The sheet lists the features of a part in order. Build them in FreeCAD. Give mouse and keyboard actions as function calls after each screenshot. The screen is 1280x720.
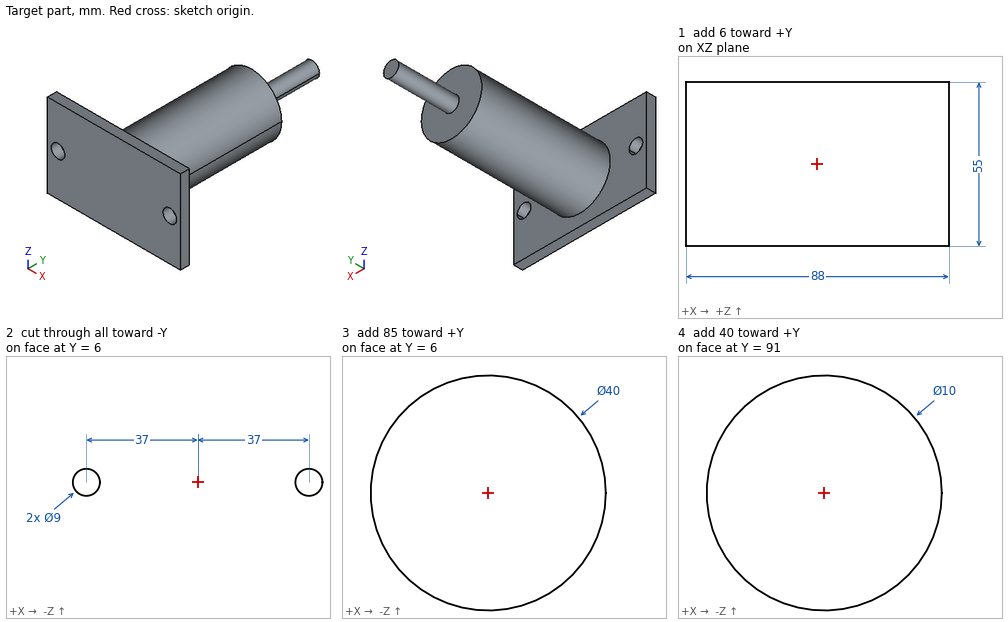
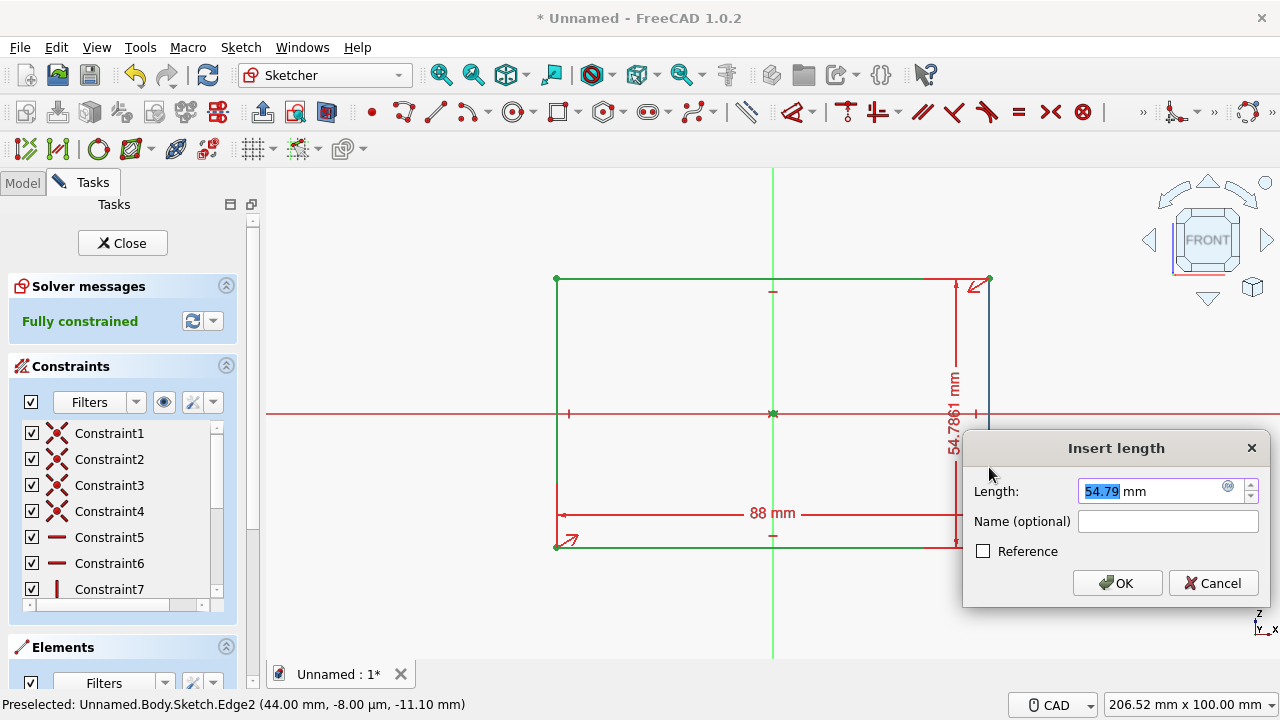
text(55)
key(Return)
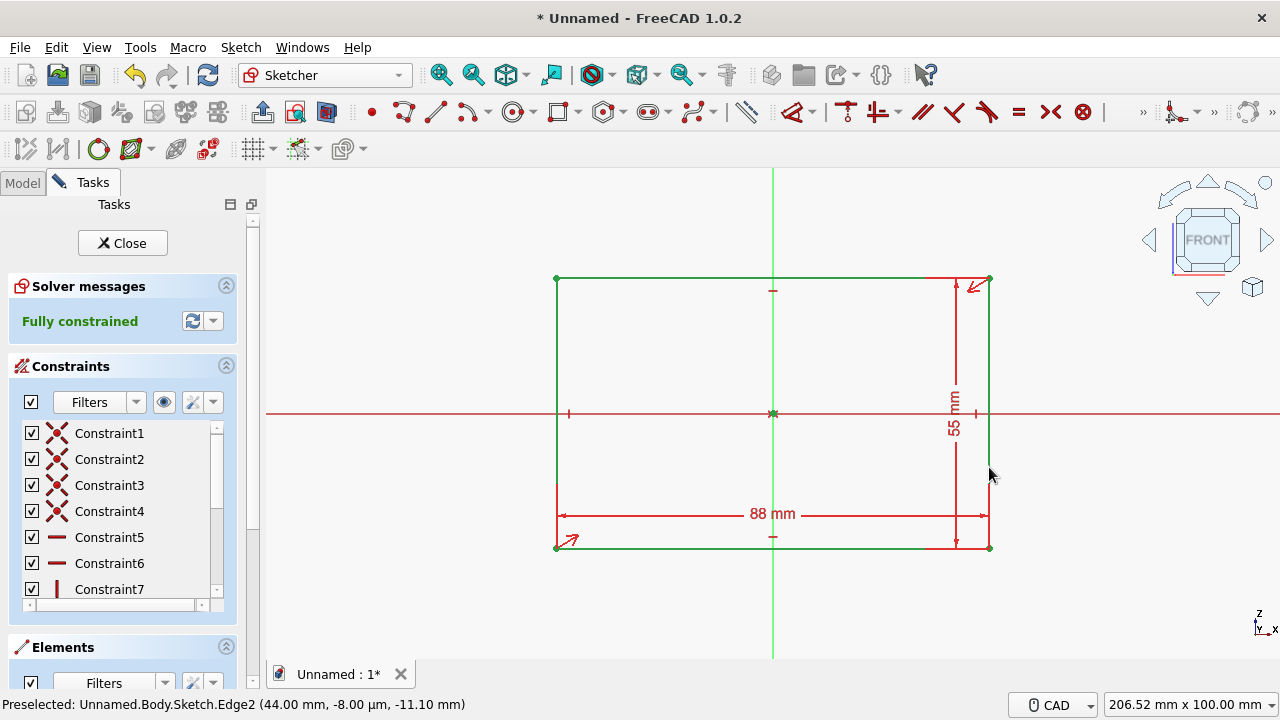
click(123, 243)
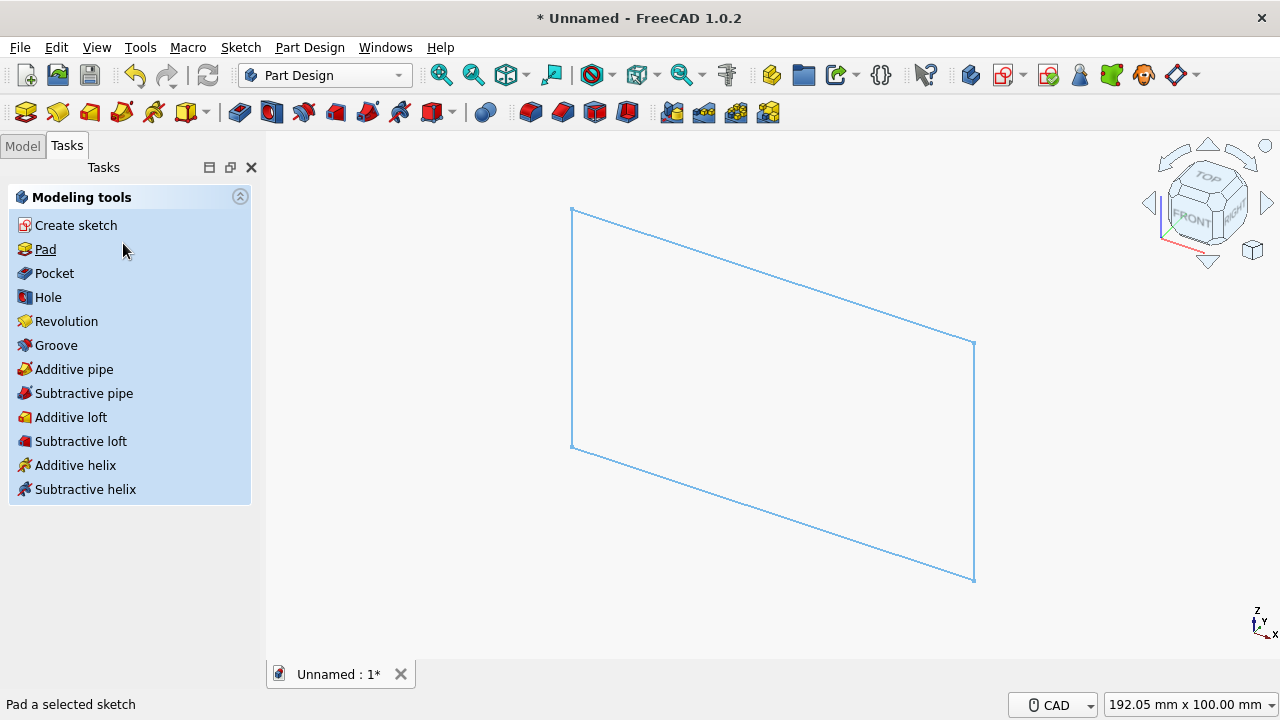
click(26, 112)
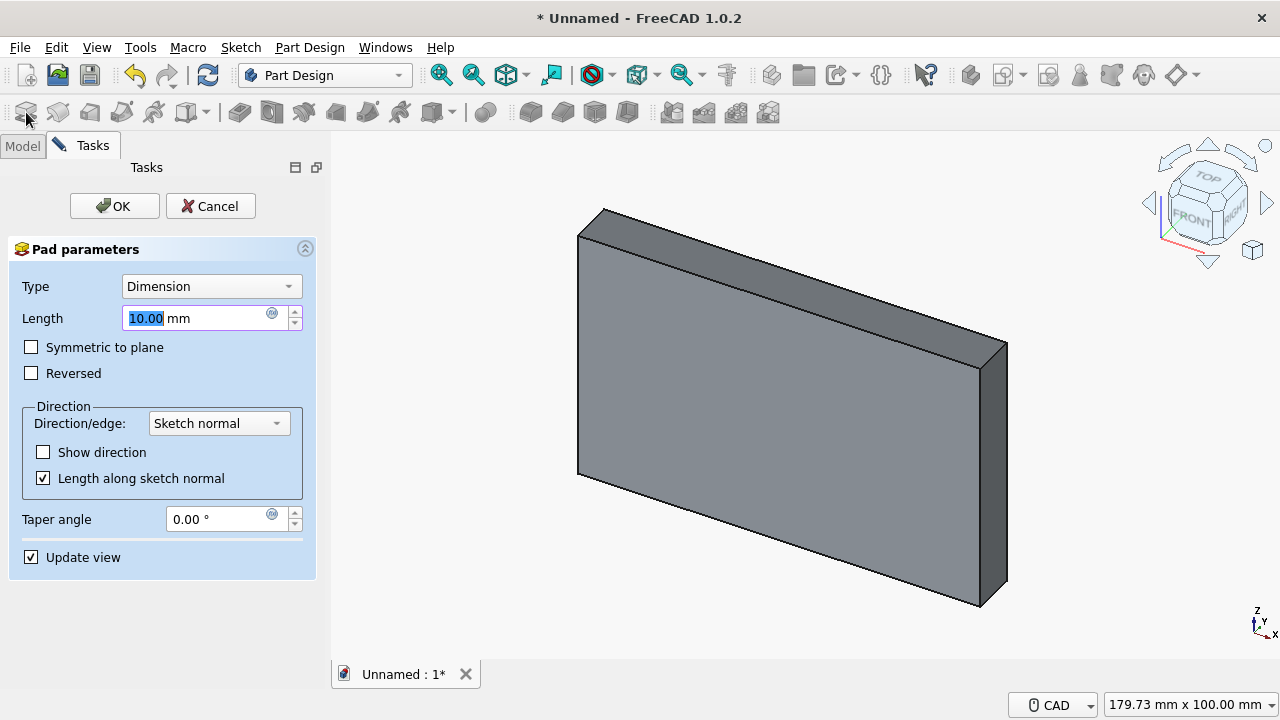
text(6)
key(Tab)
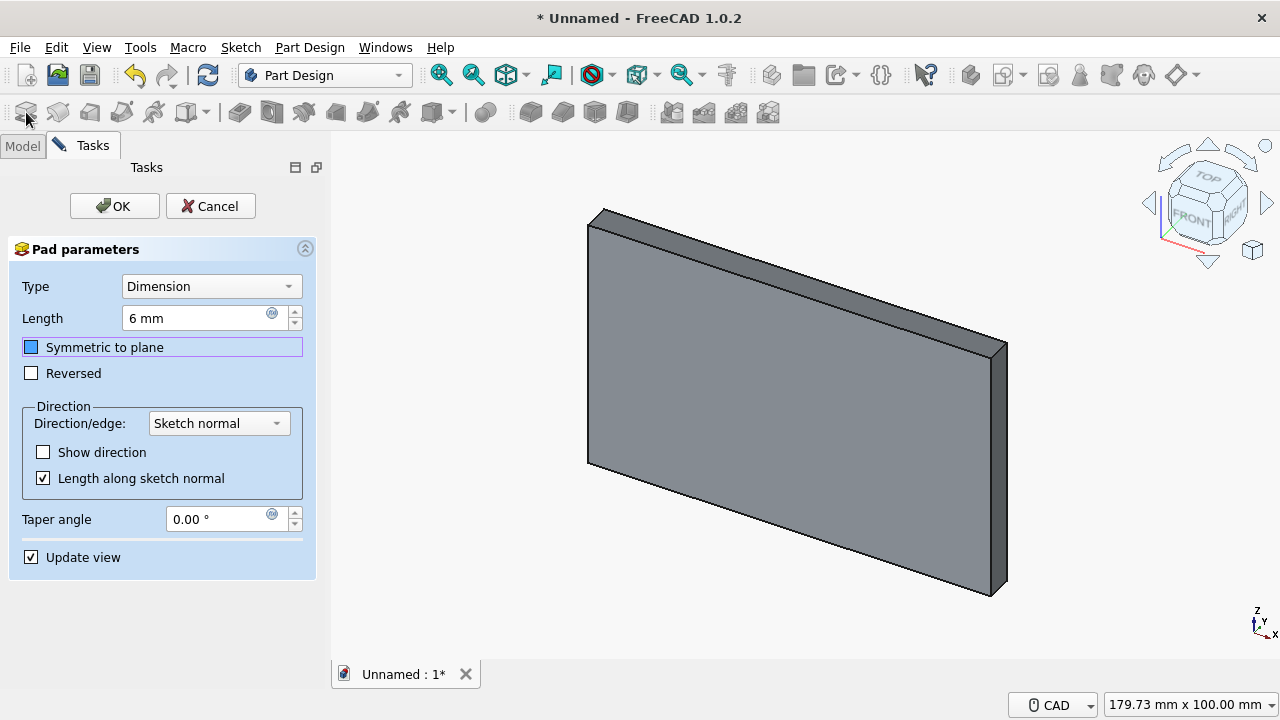
click(30, 373)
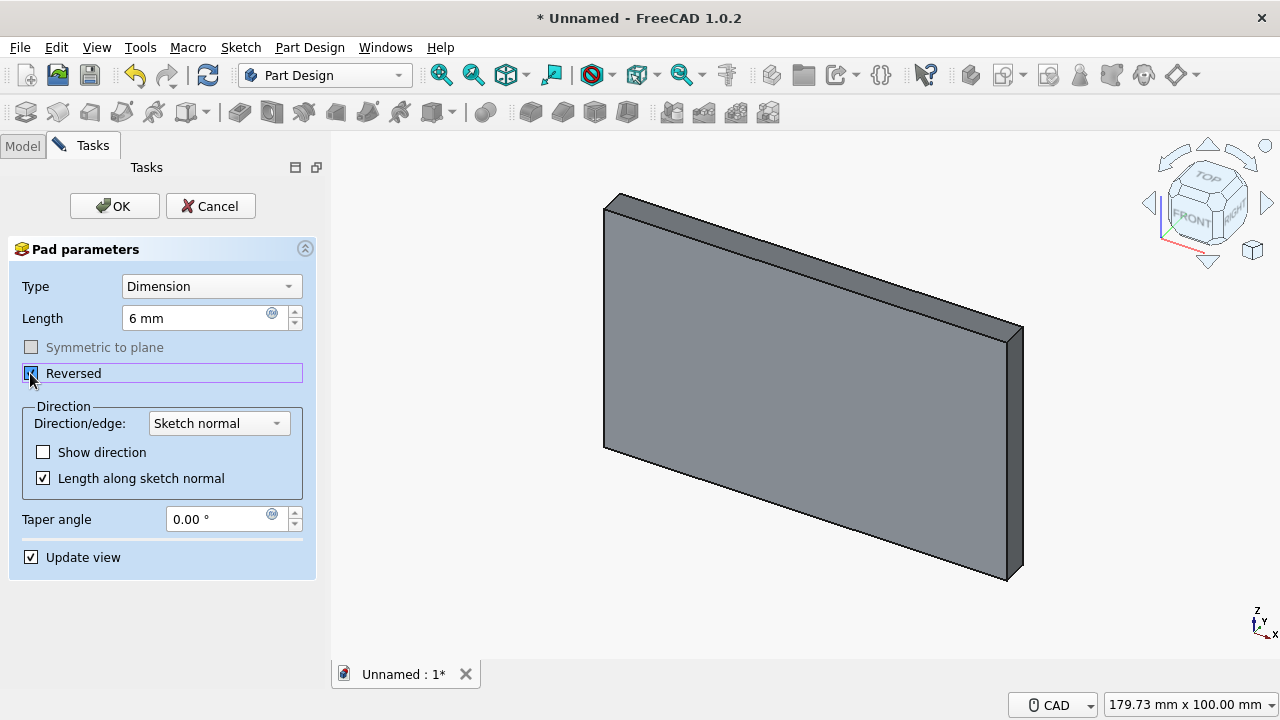
click(115, 206)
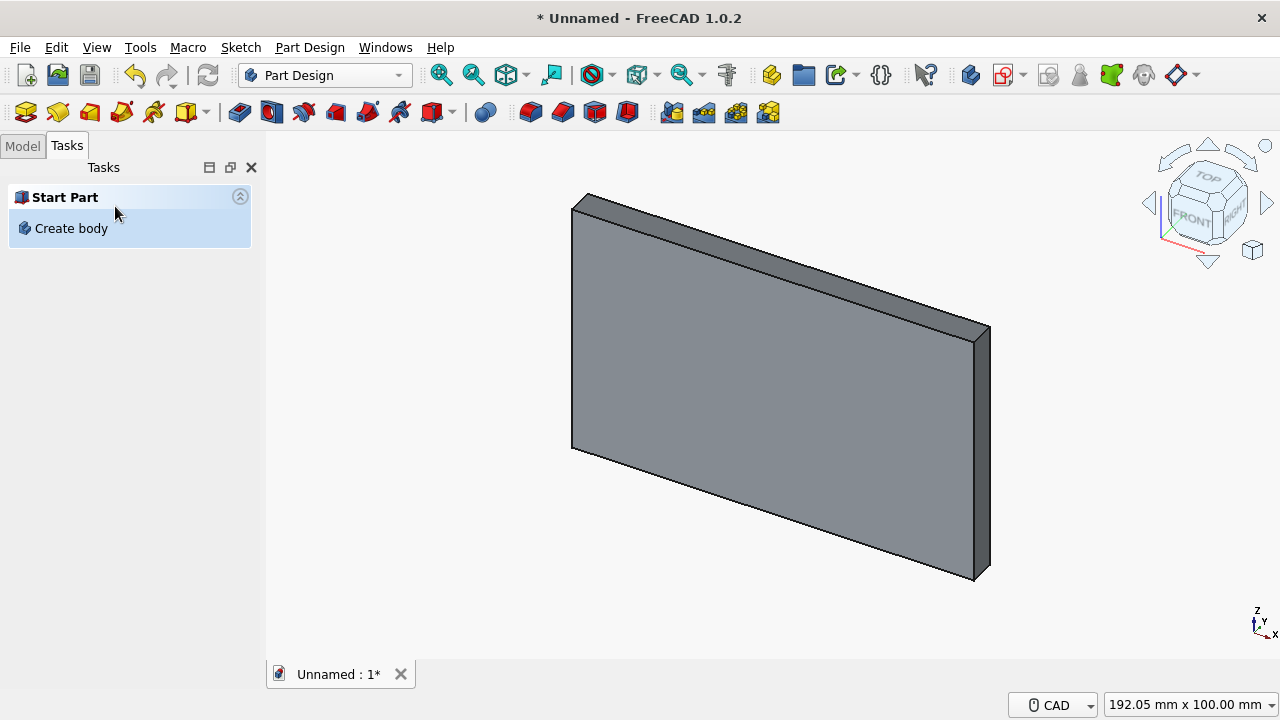
key(4)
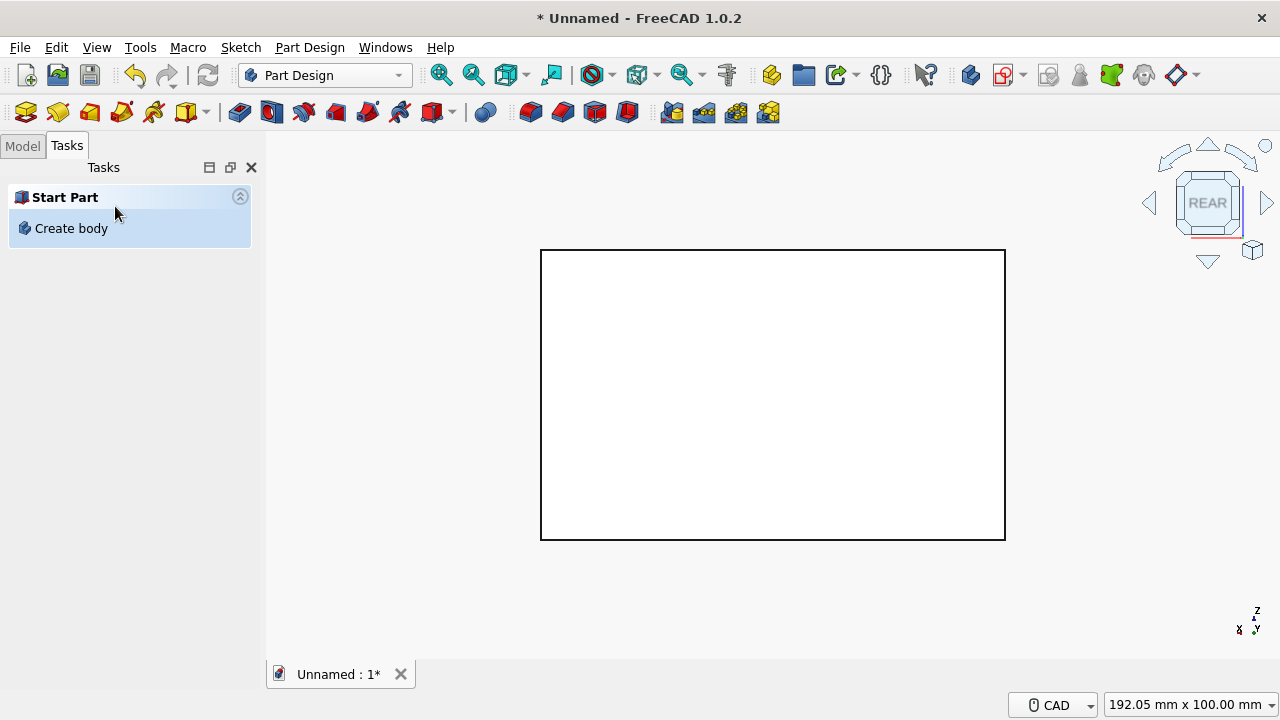
click(707, 394)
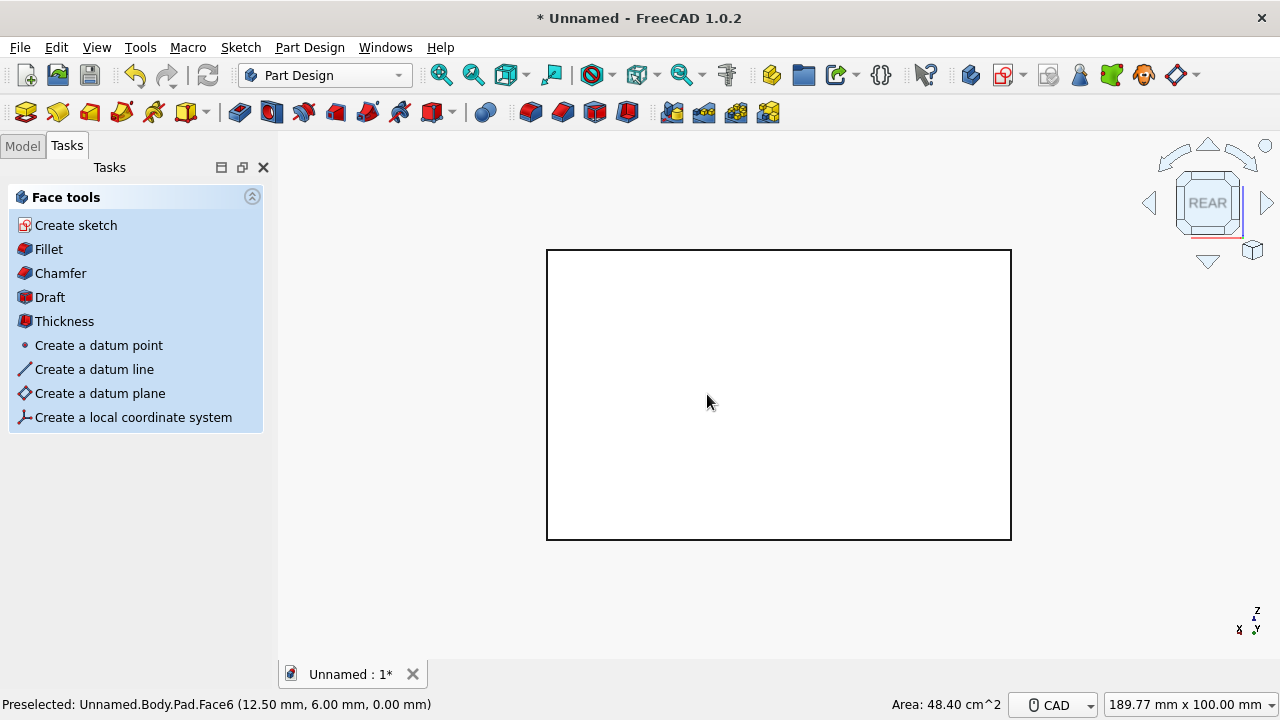
click(1004, 76)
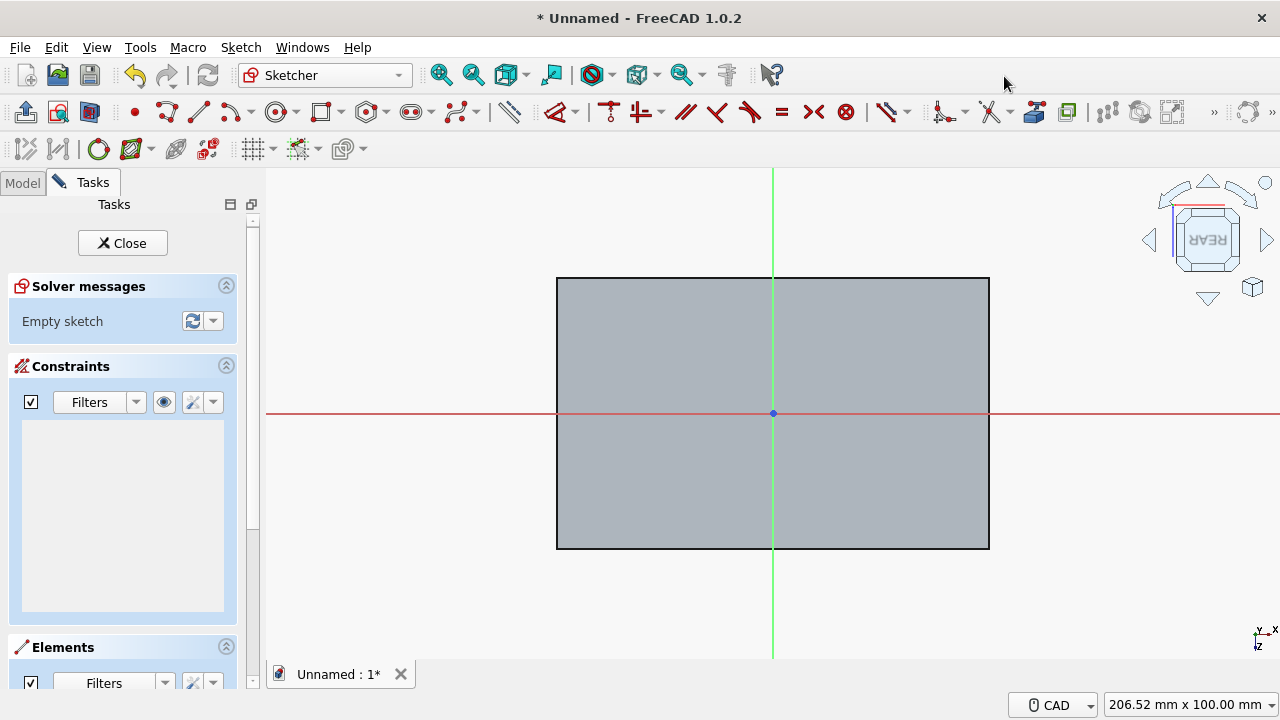
scroll(912, 414, up, 2)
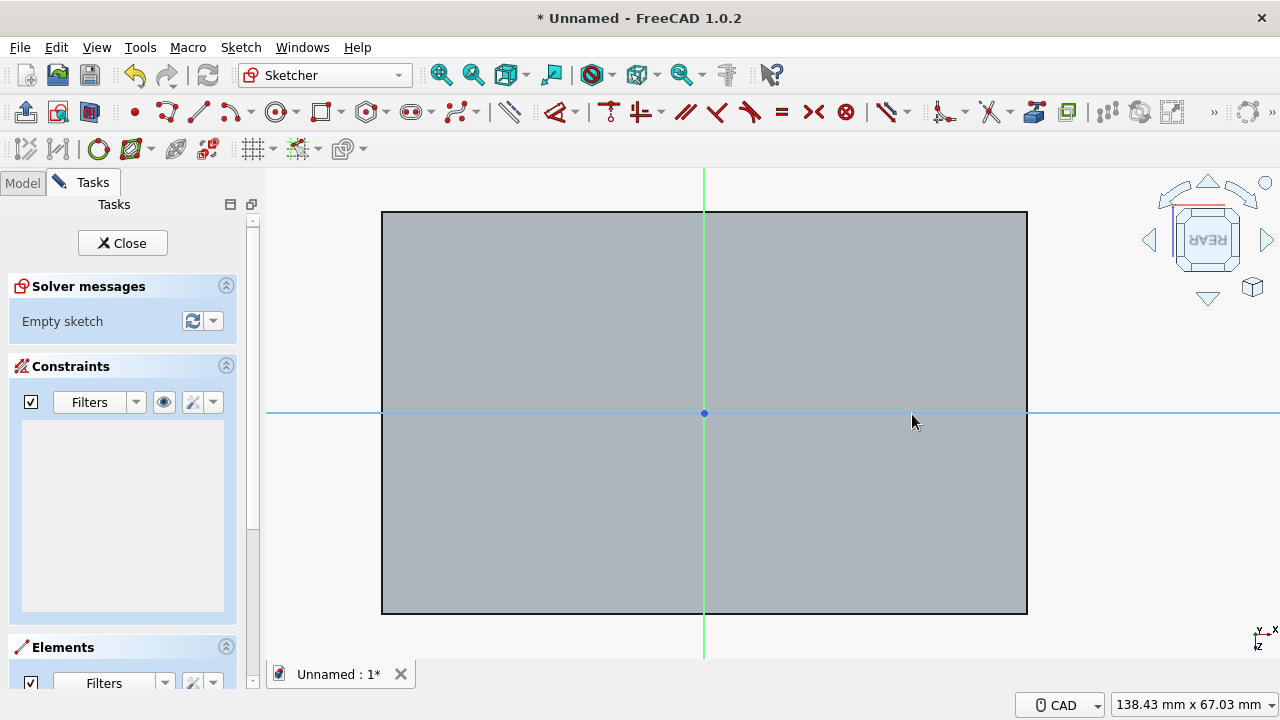
key(g)
key(c)